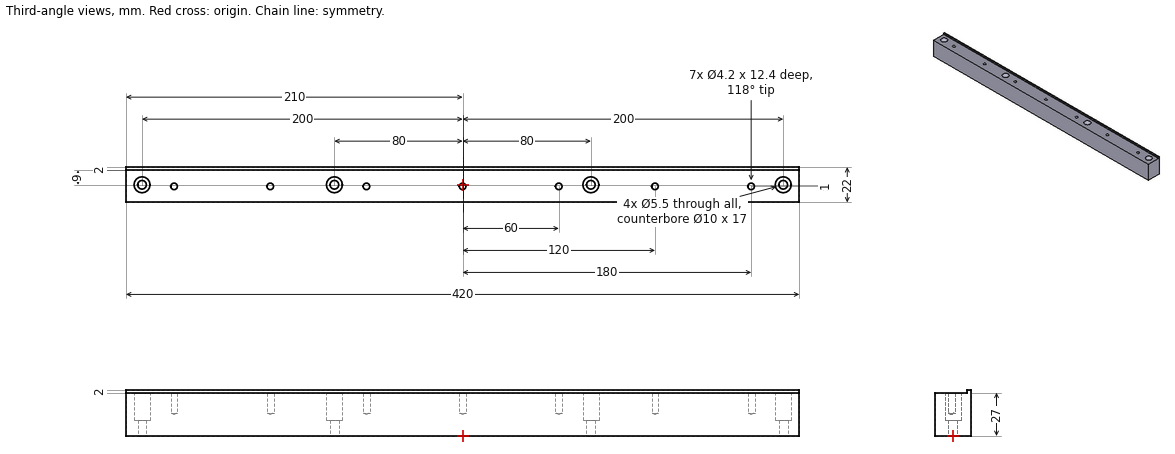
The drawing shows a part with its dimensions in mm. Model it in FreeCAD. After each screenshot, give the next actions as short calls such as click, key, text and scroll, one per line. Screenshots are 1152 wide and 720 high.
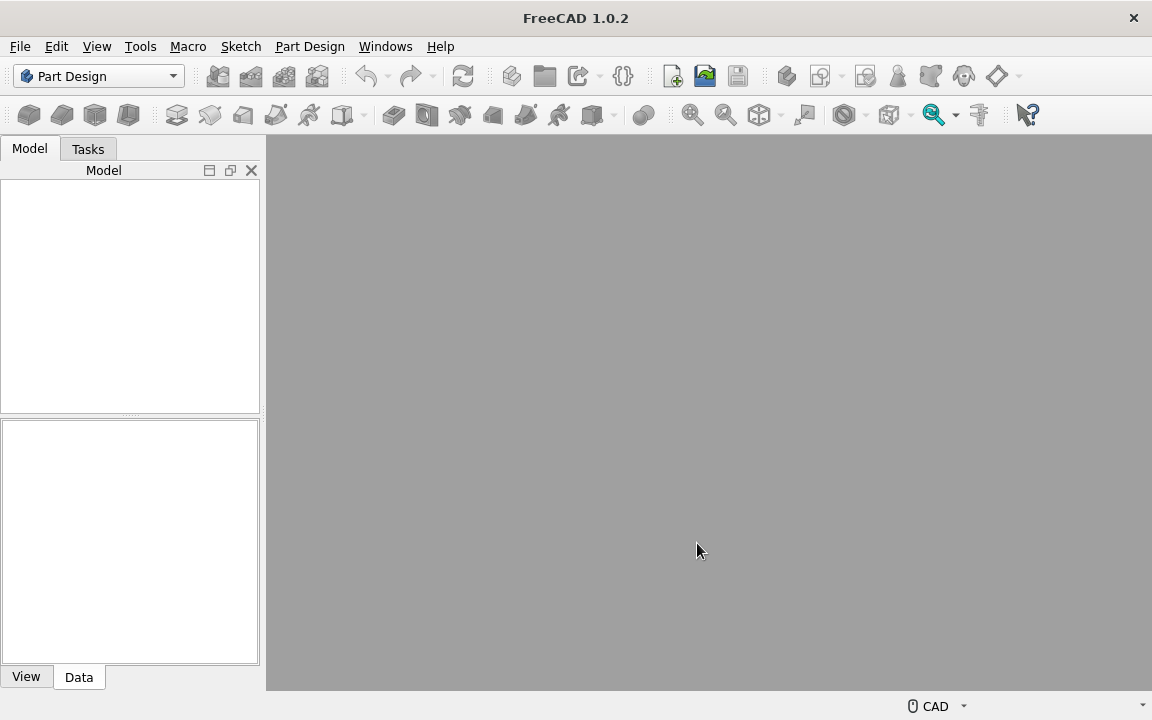
click(672, 76)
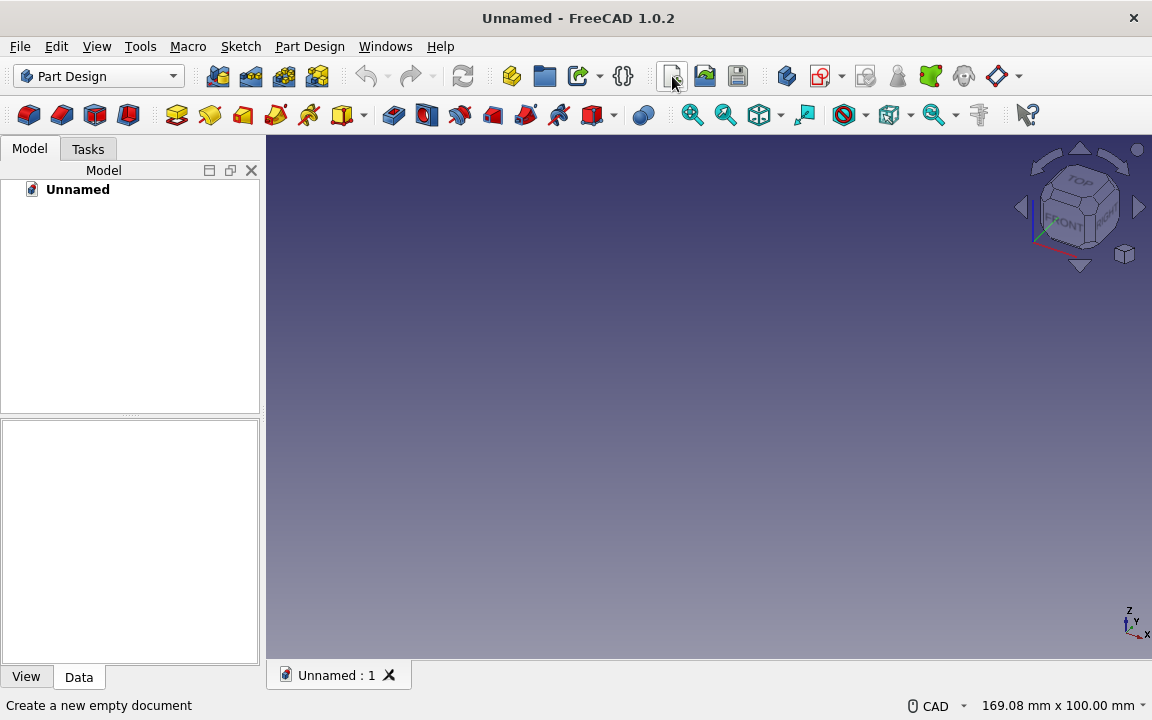
click(820, 76)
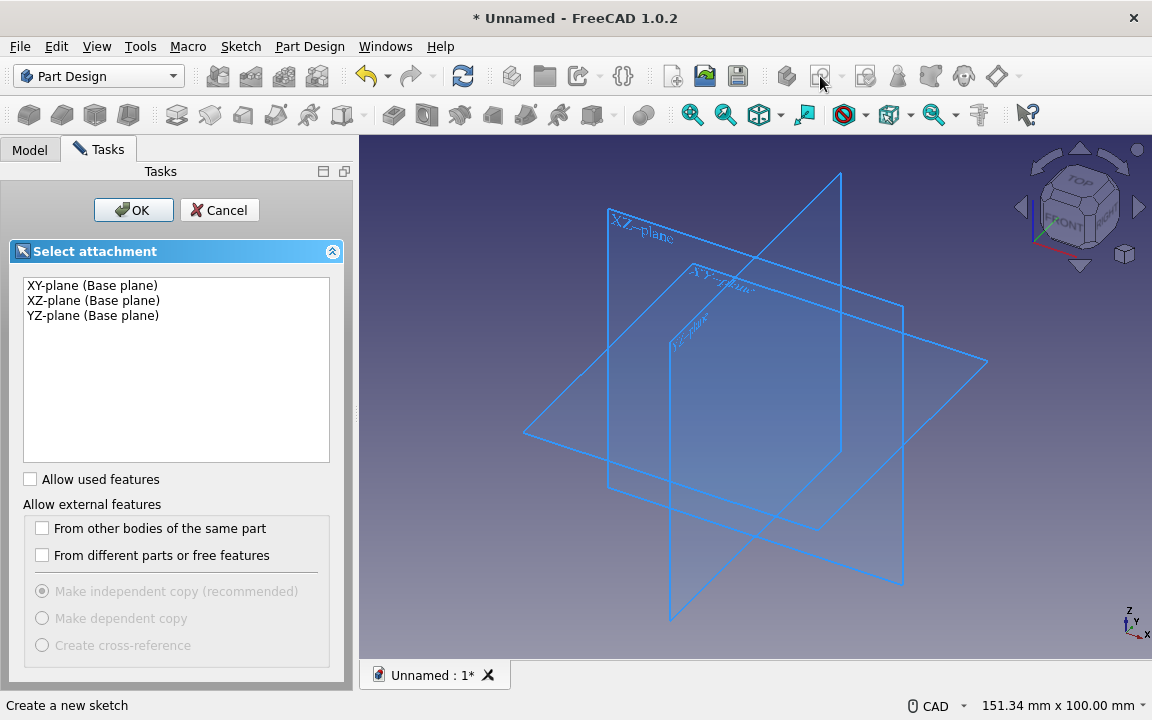
click(84, 286)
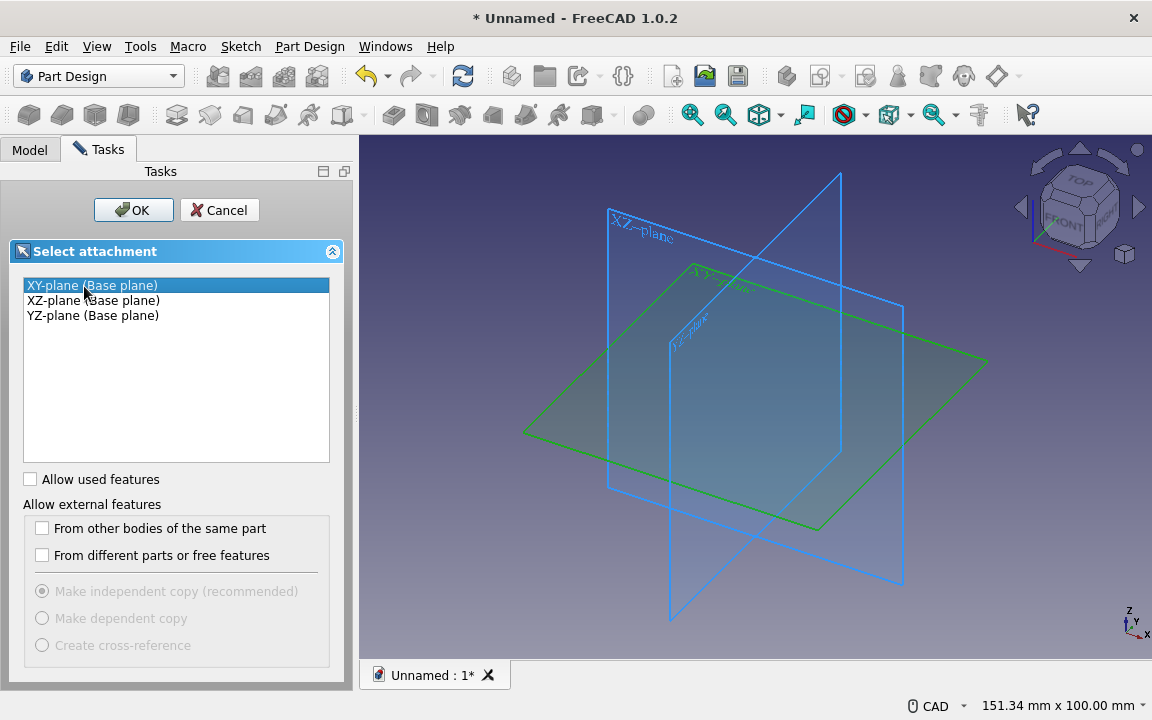
click(134, 210)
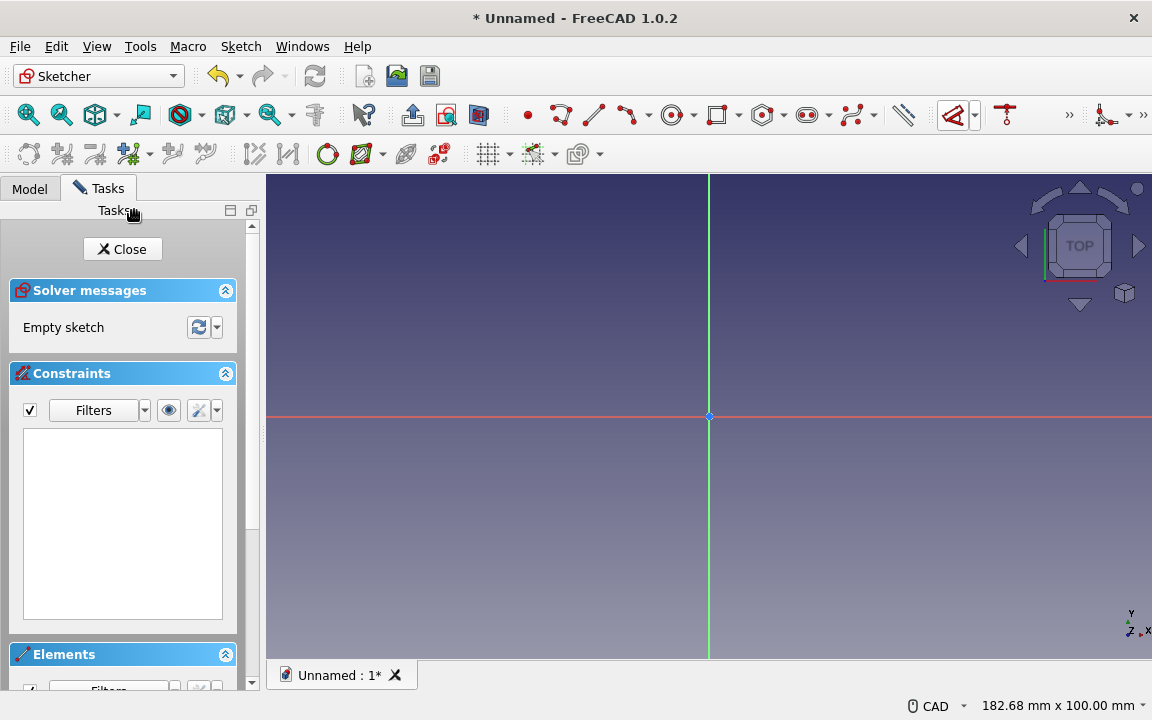
scroll(618, 417, down, 7)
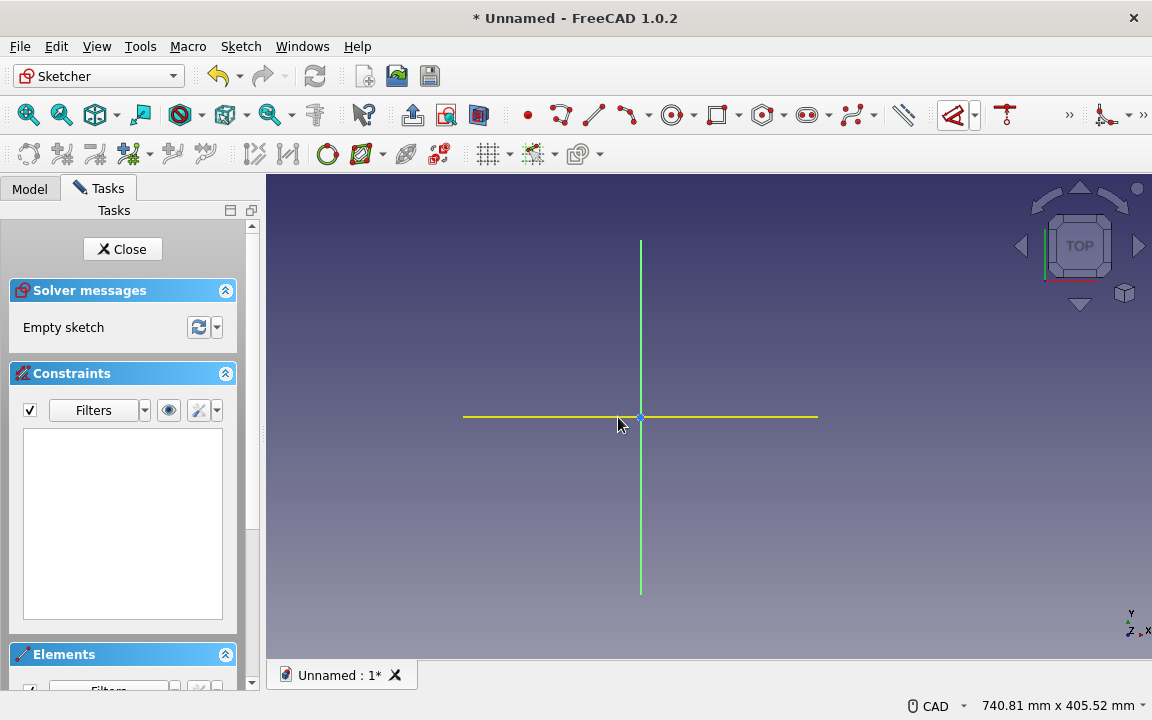
key(g)
key(v)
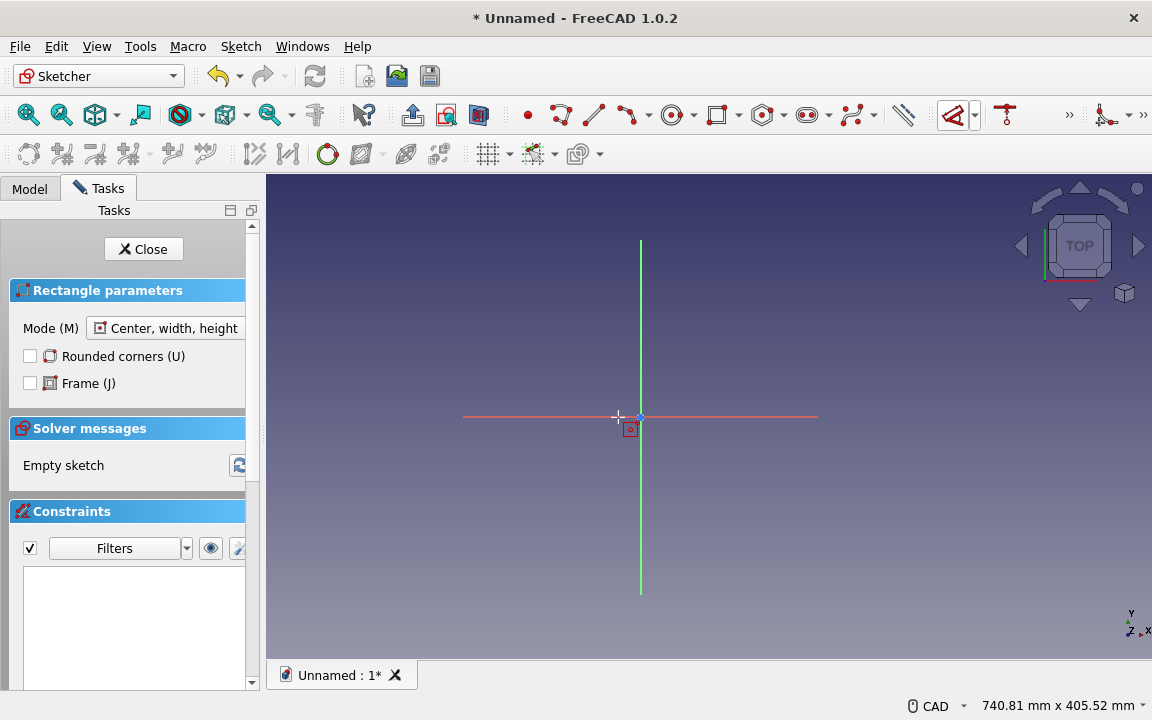
click(641, 417)
move(892, 404)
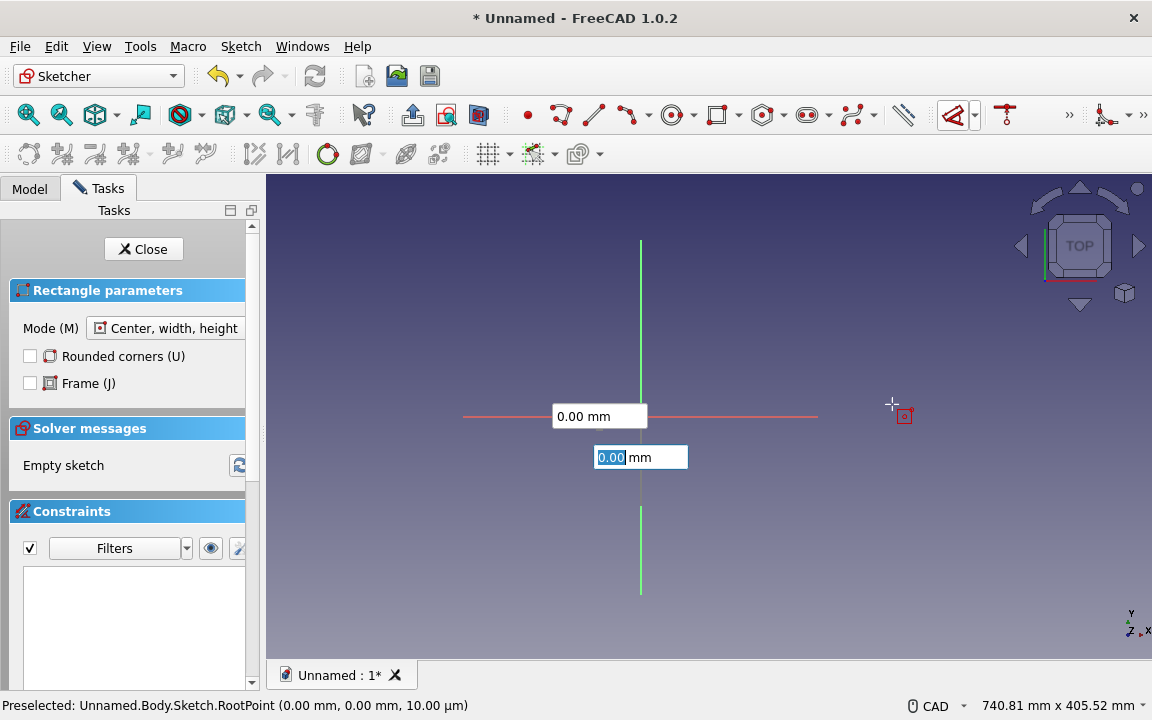
text(420)
key(Tab)
text(22)
key(Return)
key(Escape)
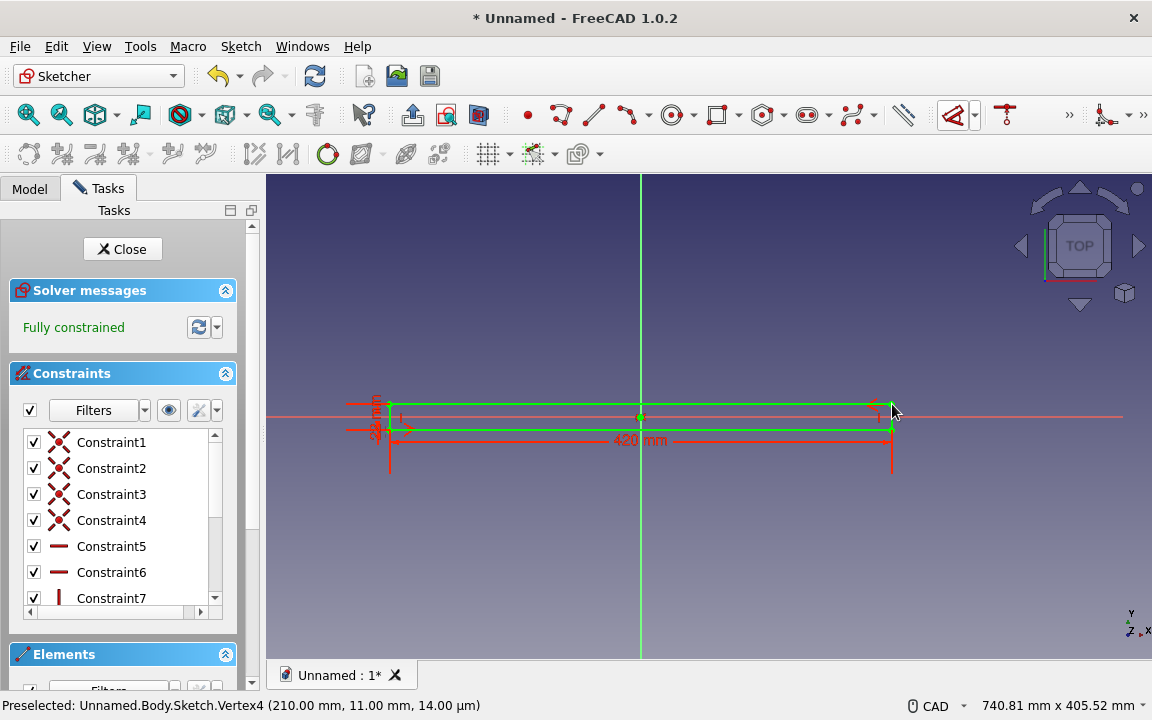
click(123, 249)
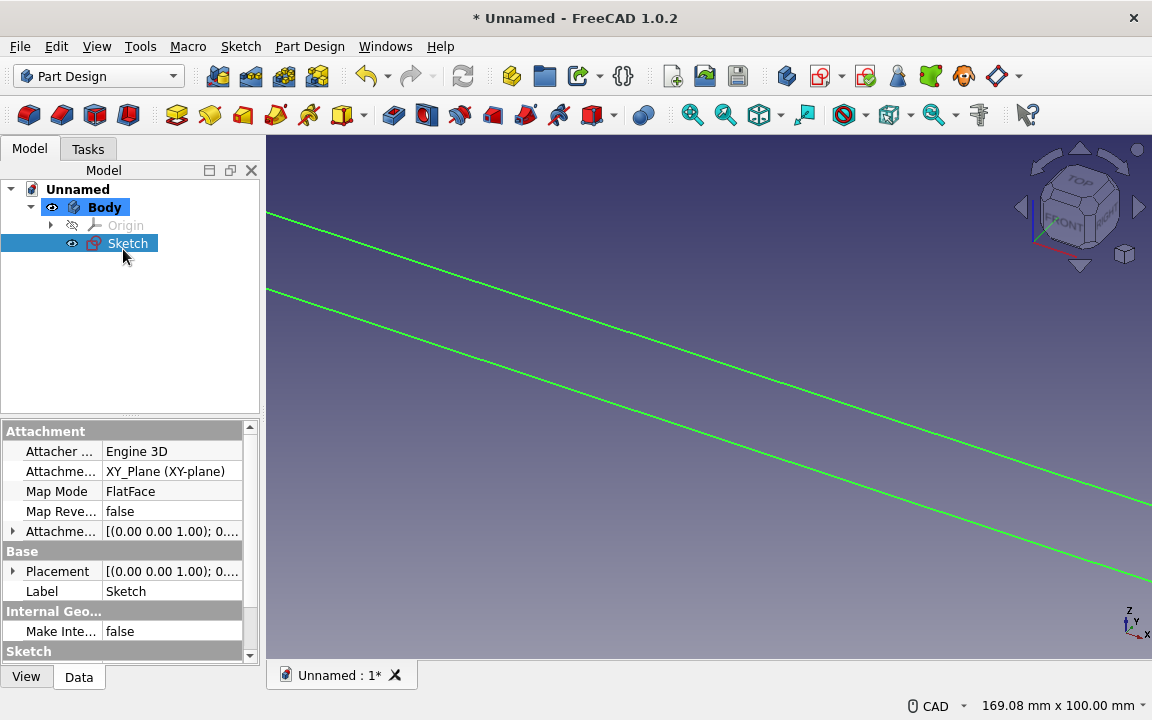
click(177, 116)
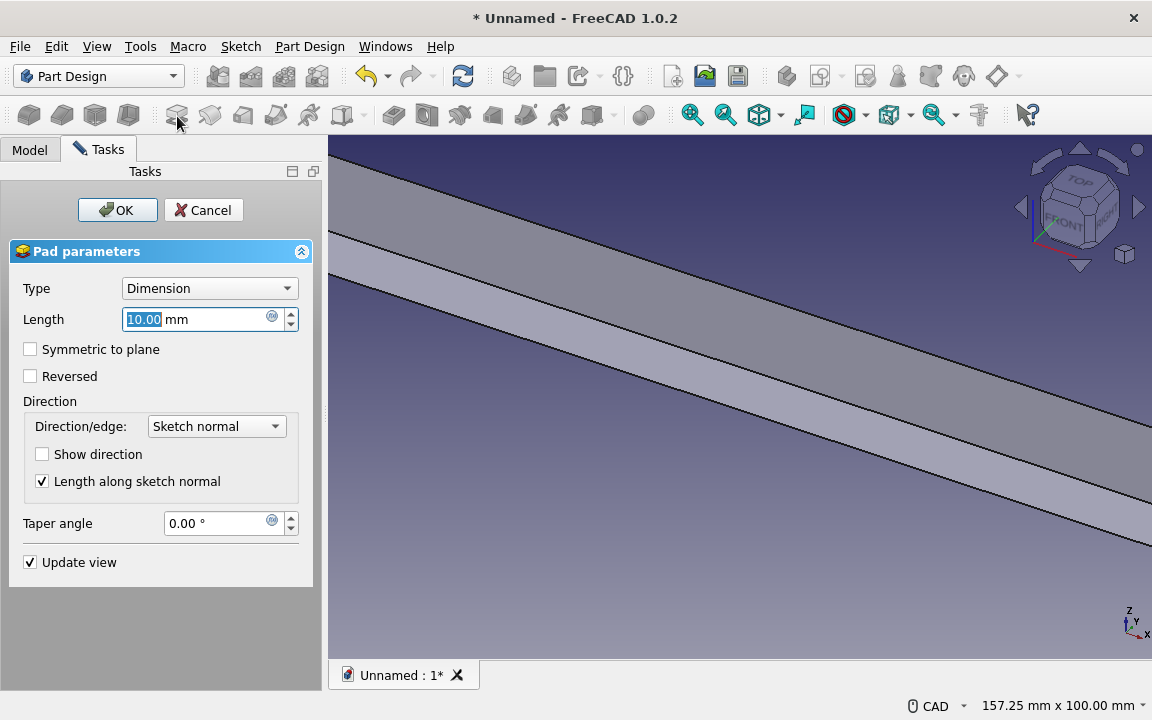
text(27)
key(Tab)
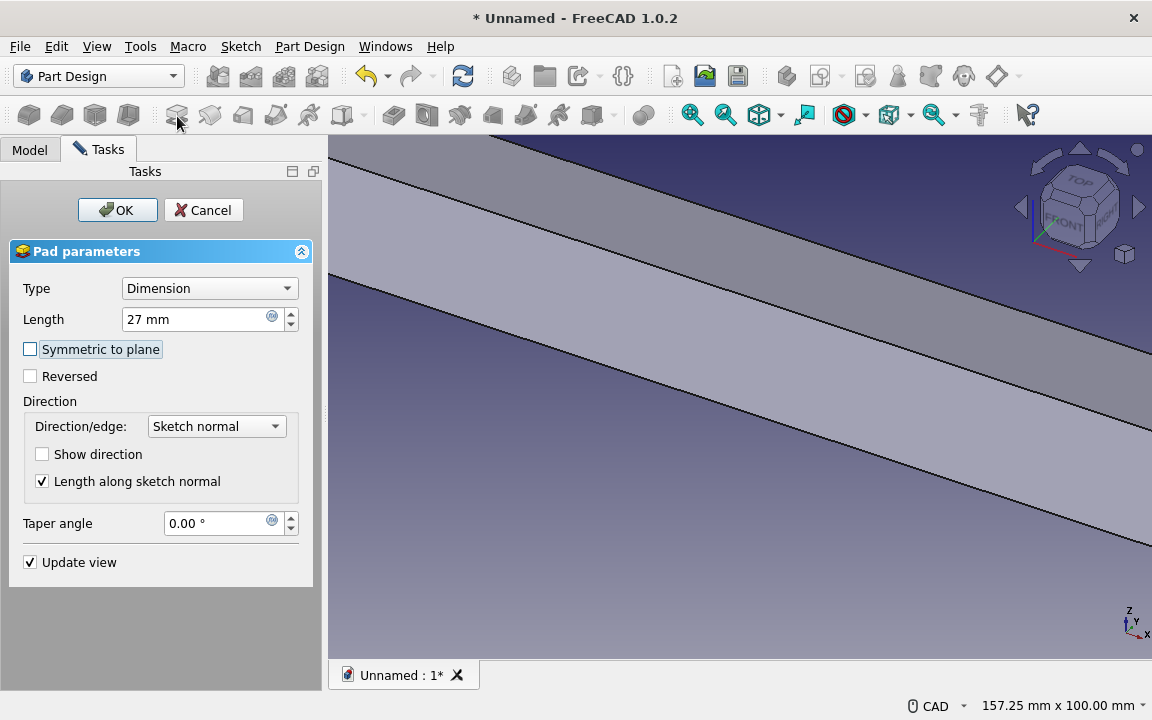
click(118, 210)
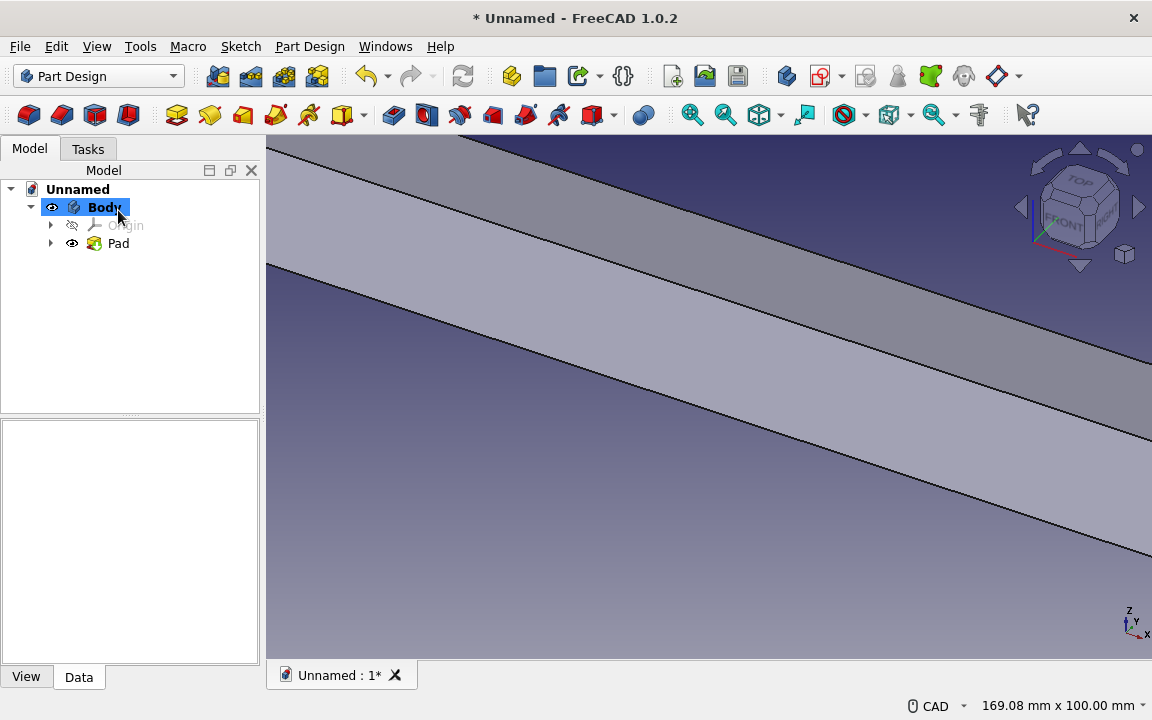
key(v)
key(f)